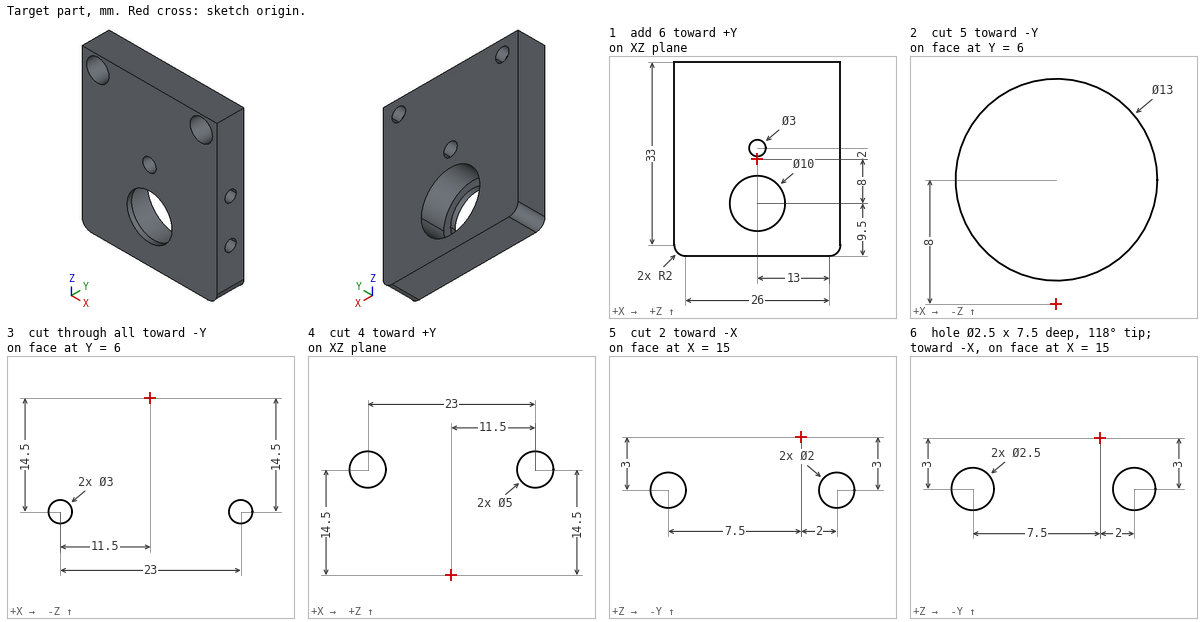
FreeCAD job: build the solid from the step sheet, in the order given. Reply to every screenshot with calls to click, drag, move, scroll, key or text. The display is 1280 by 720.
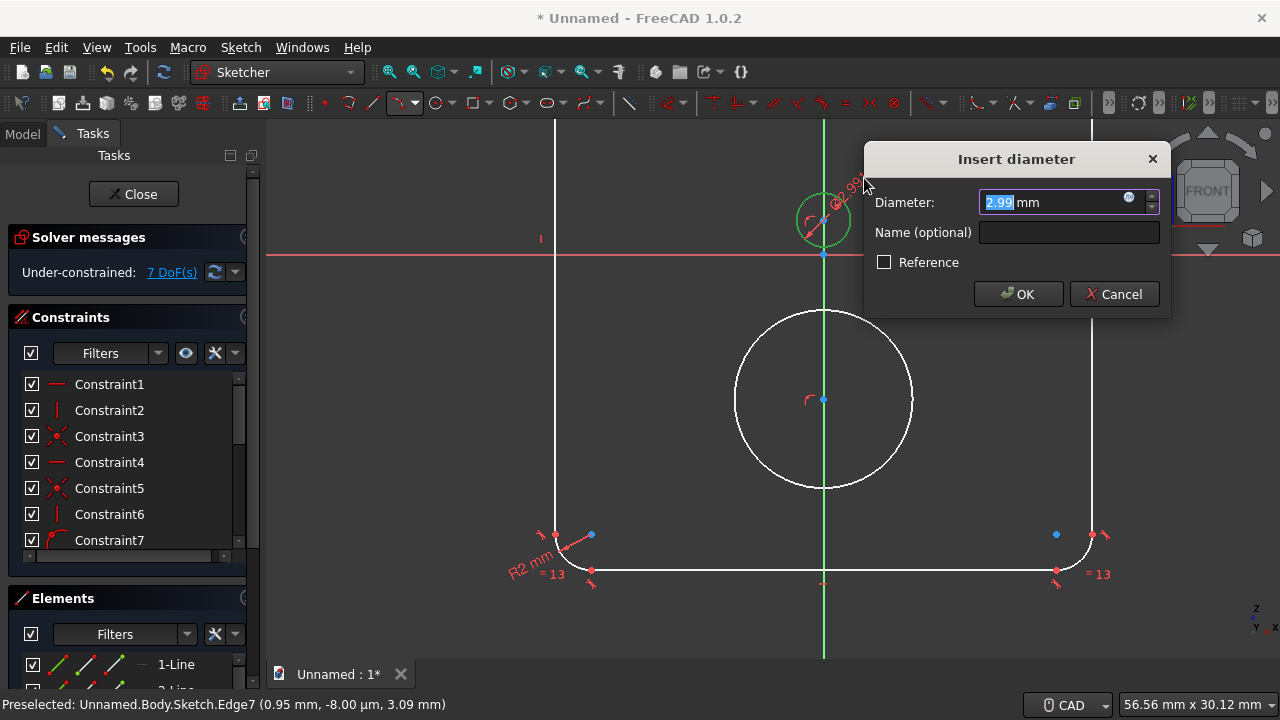
text(3)
key(Return)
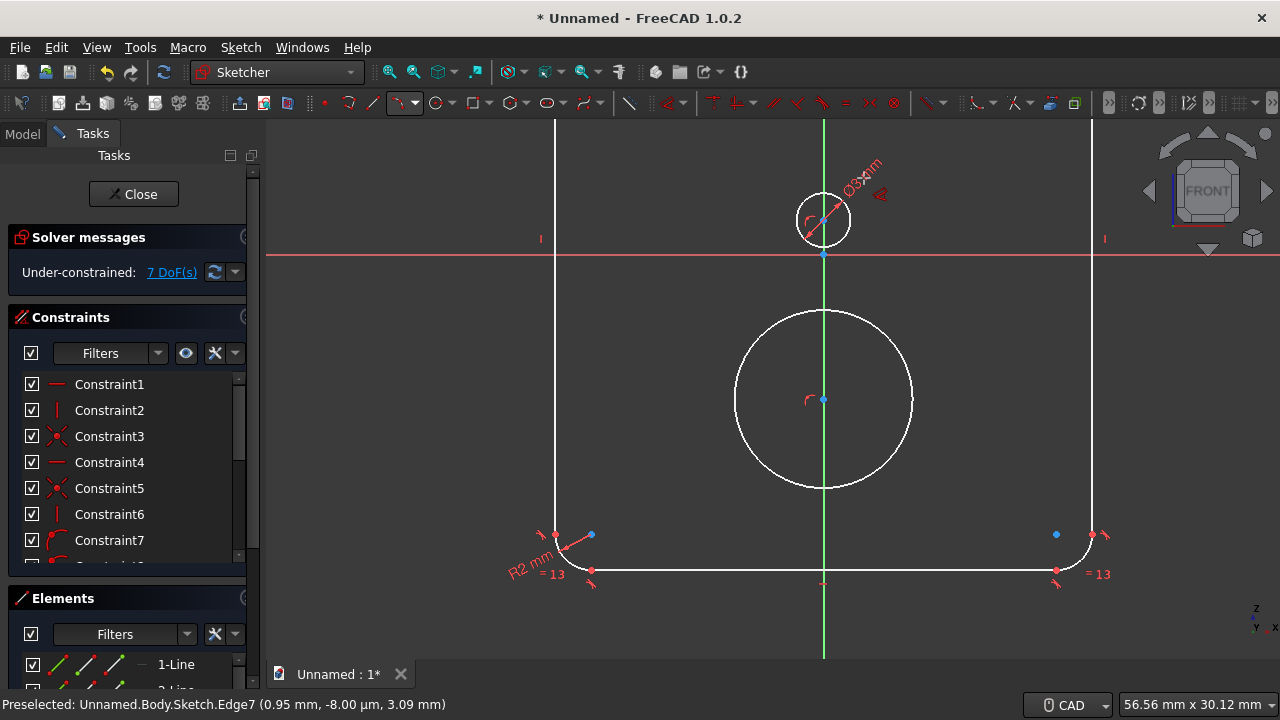
click(886, 336)
click(909, 313)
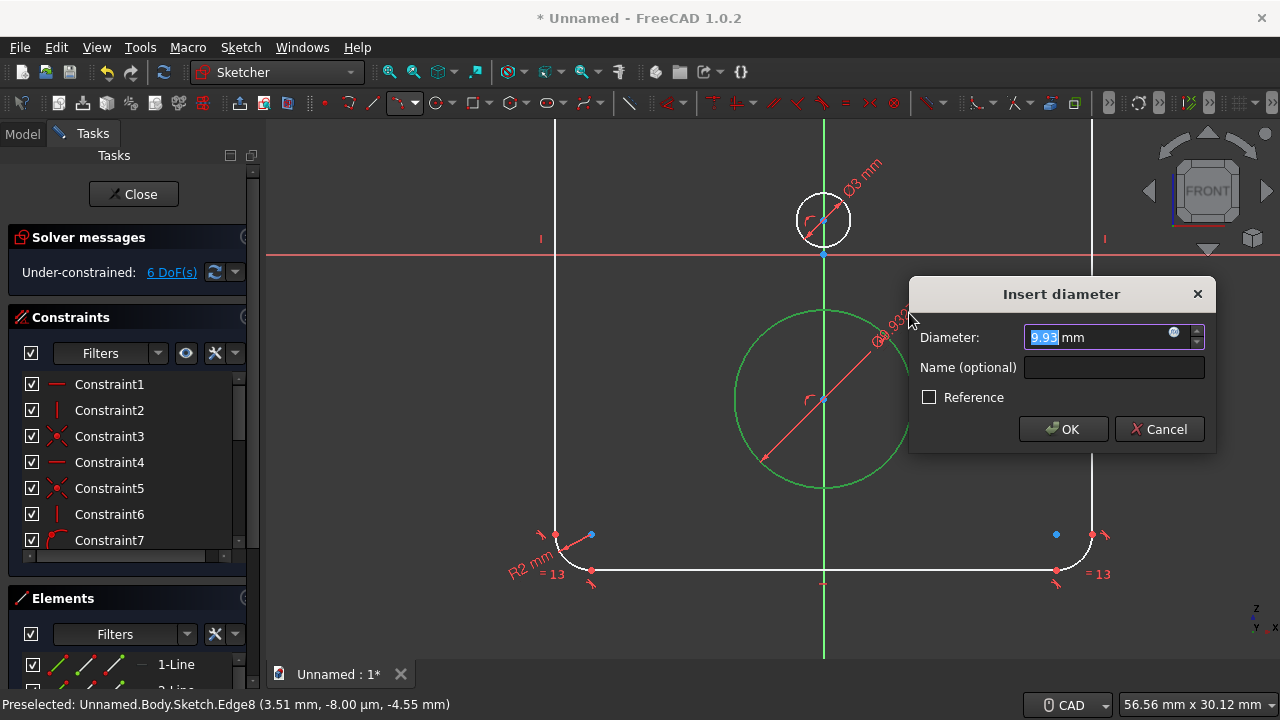
text(10)
key(Return)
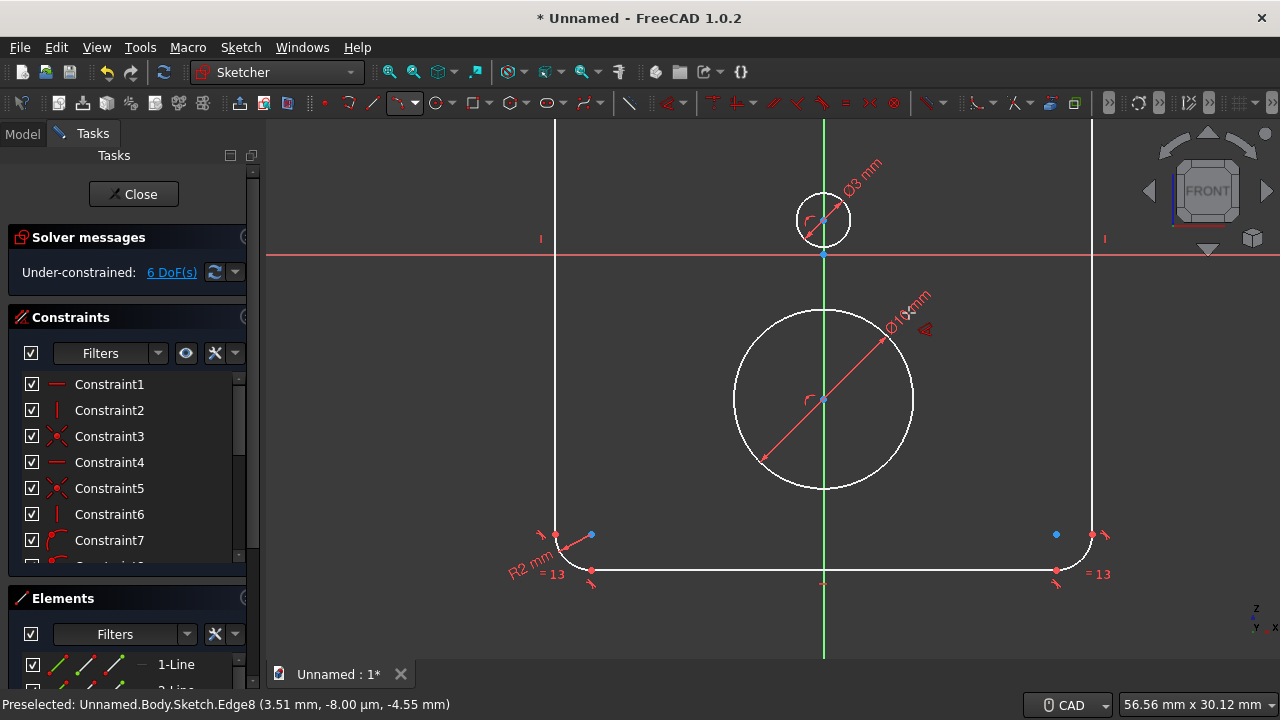
click(824, 220)
click(882, 237)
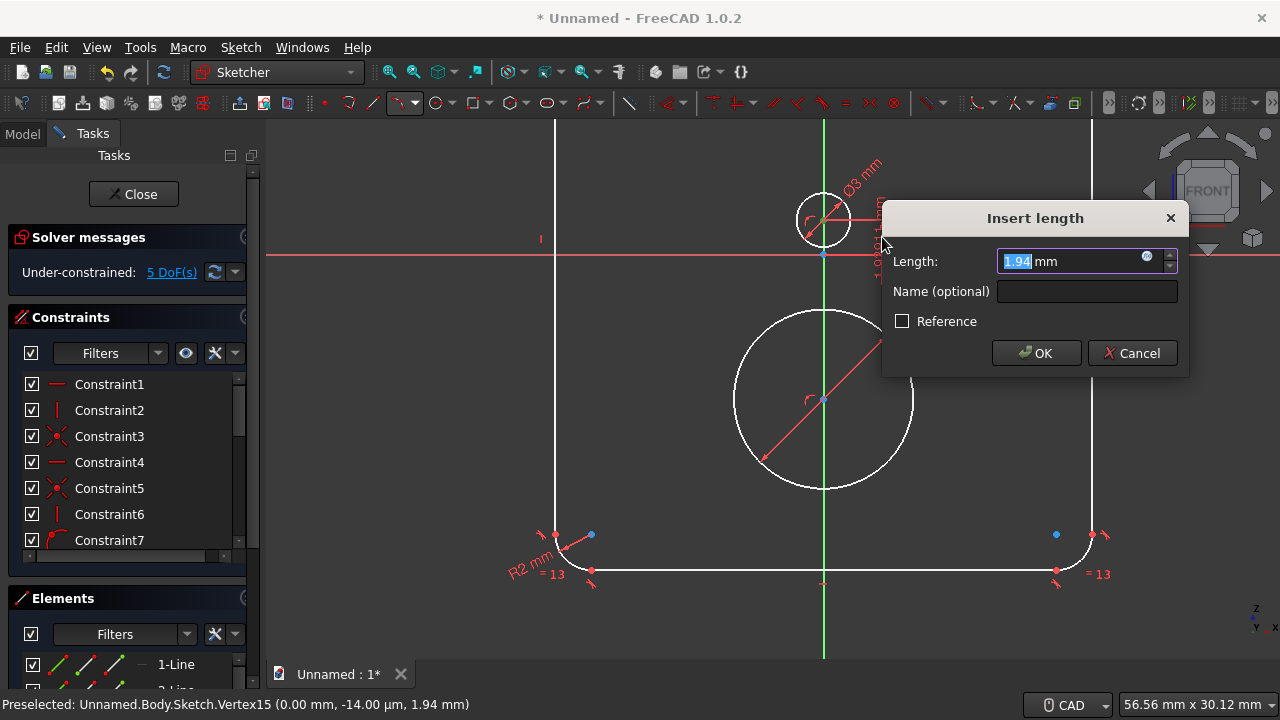
text(2)
key(Return)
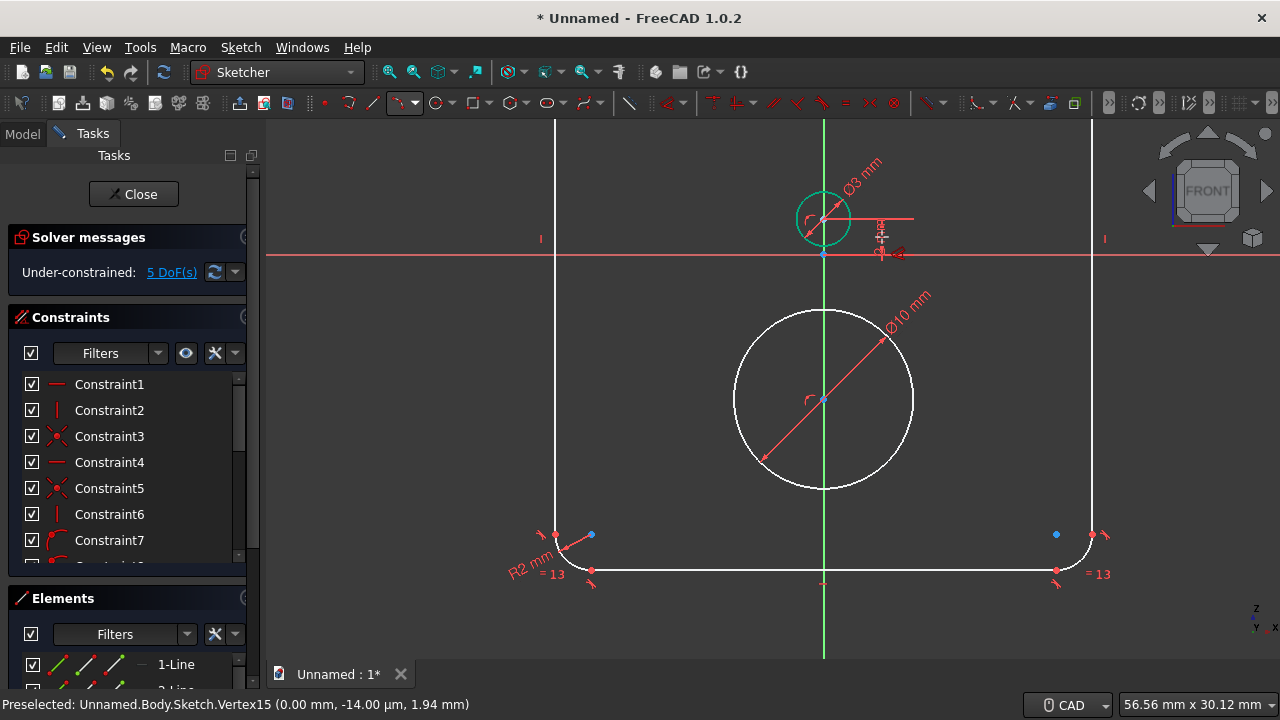
click(824, 399)
click(858, 360)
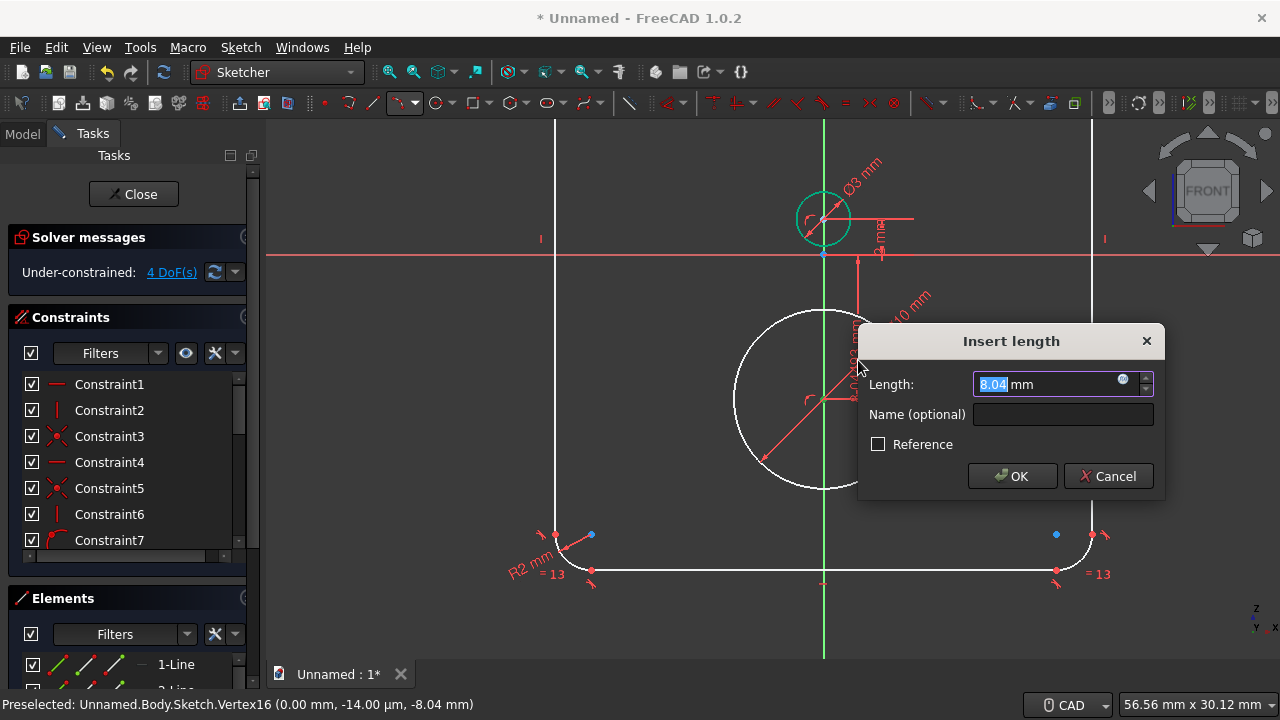
text(8)
key(Return)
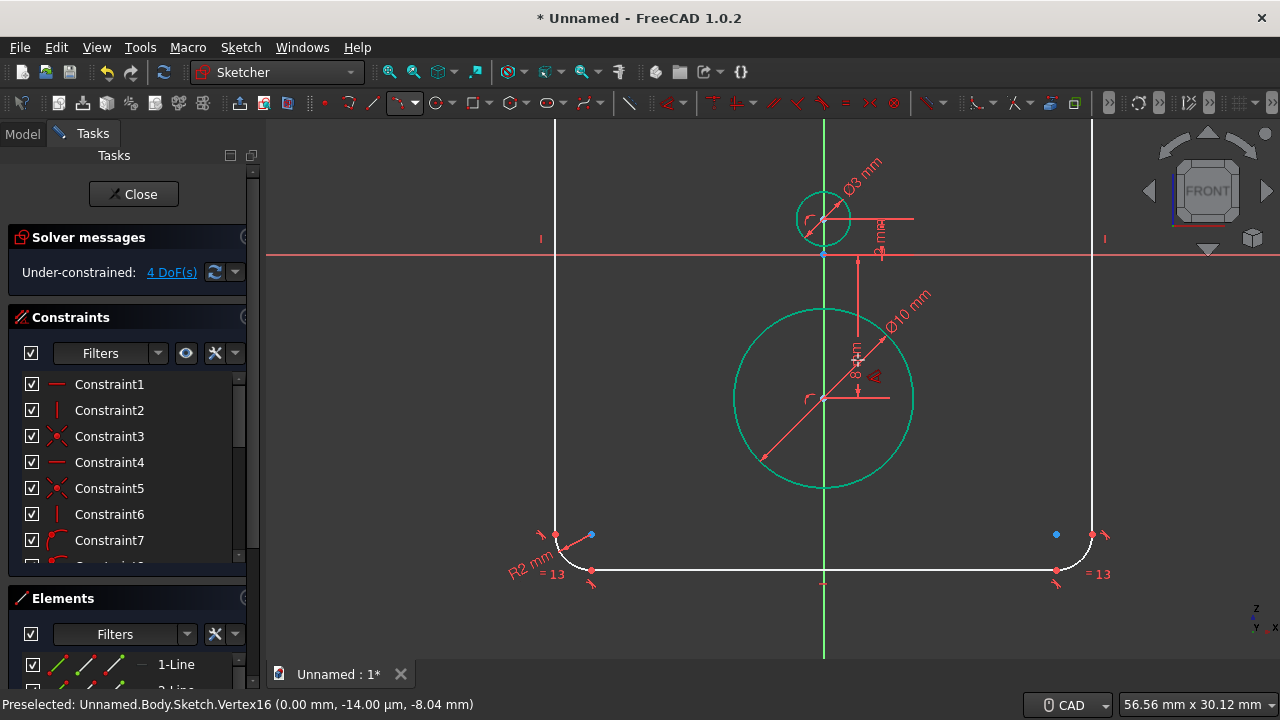
click(917, 570)
click(717, 604)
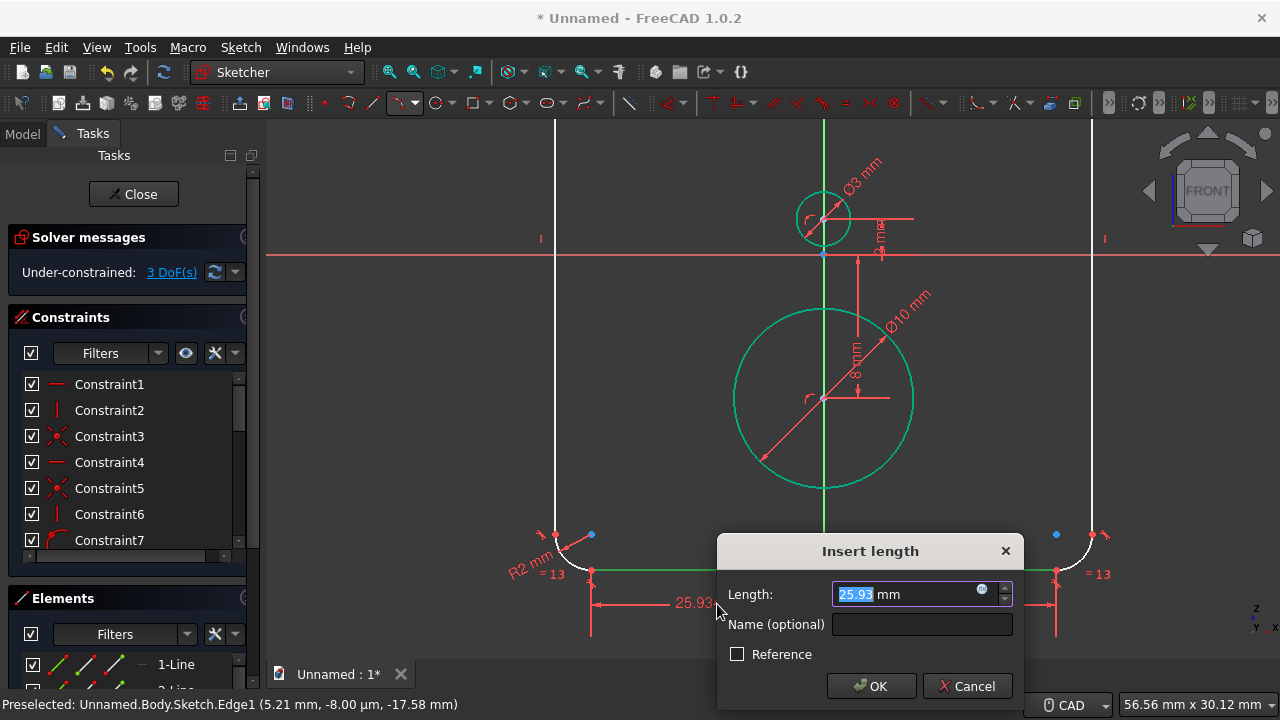
text(26)
key(Return)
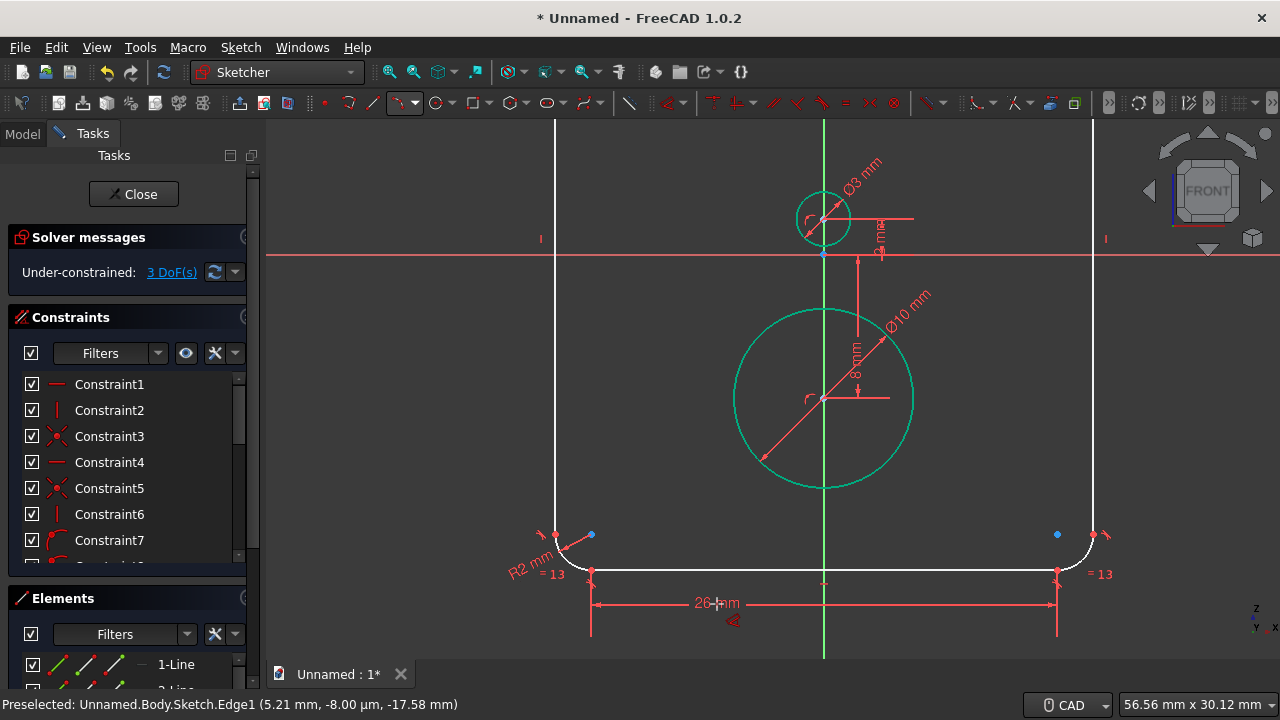
click(555, 357)
click(521, 341)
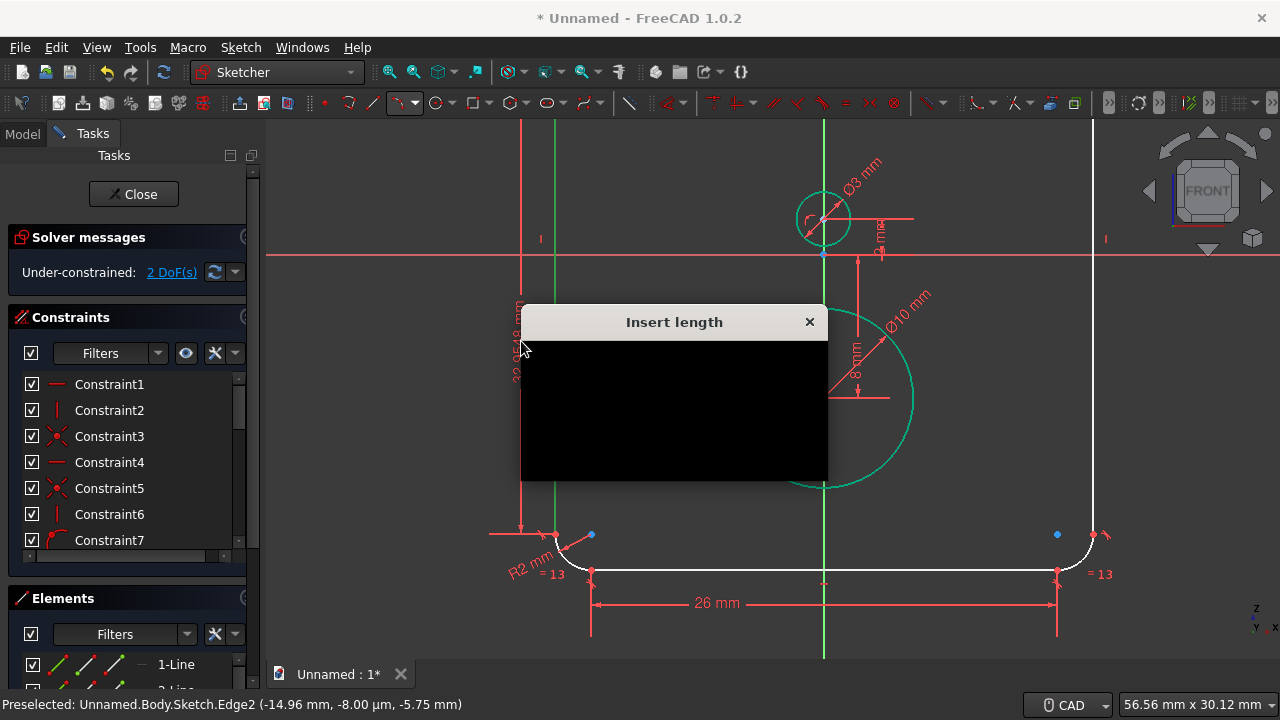
text(33)
key(Return)